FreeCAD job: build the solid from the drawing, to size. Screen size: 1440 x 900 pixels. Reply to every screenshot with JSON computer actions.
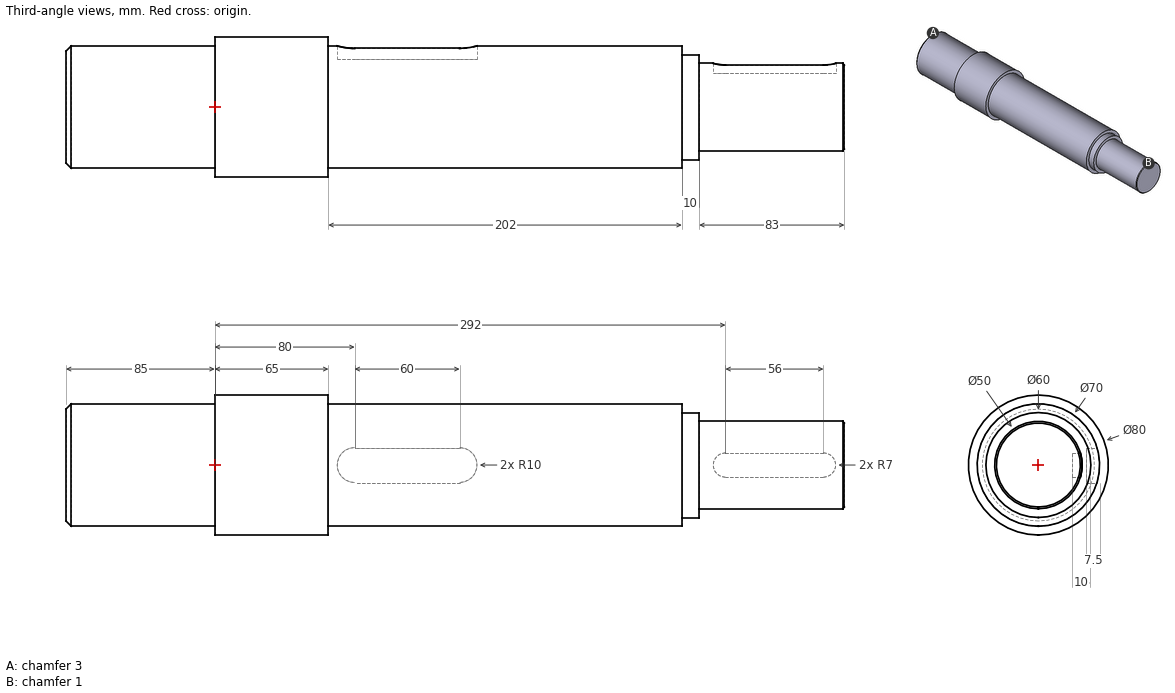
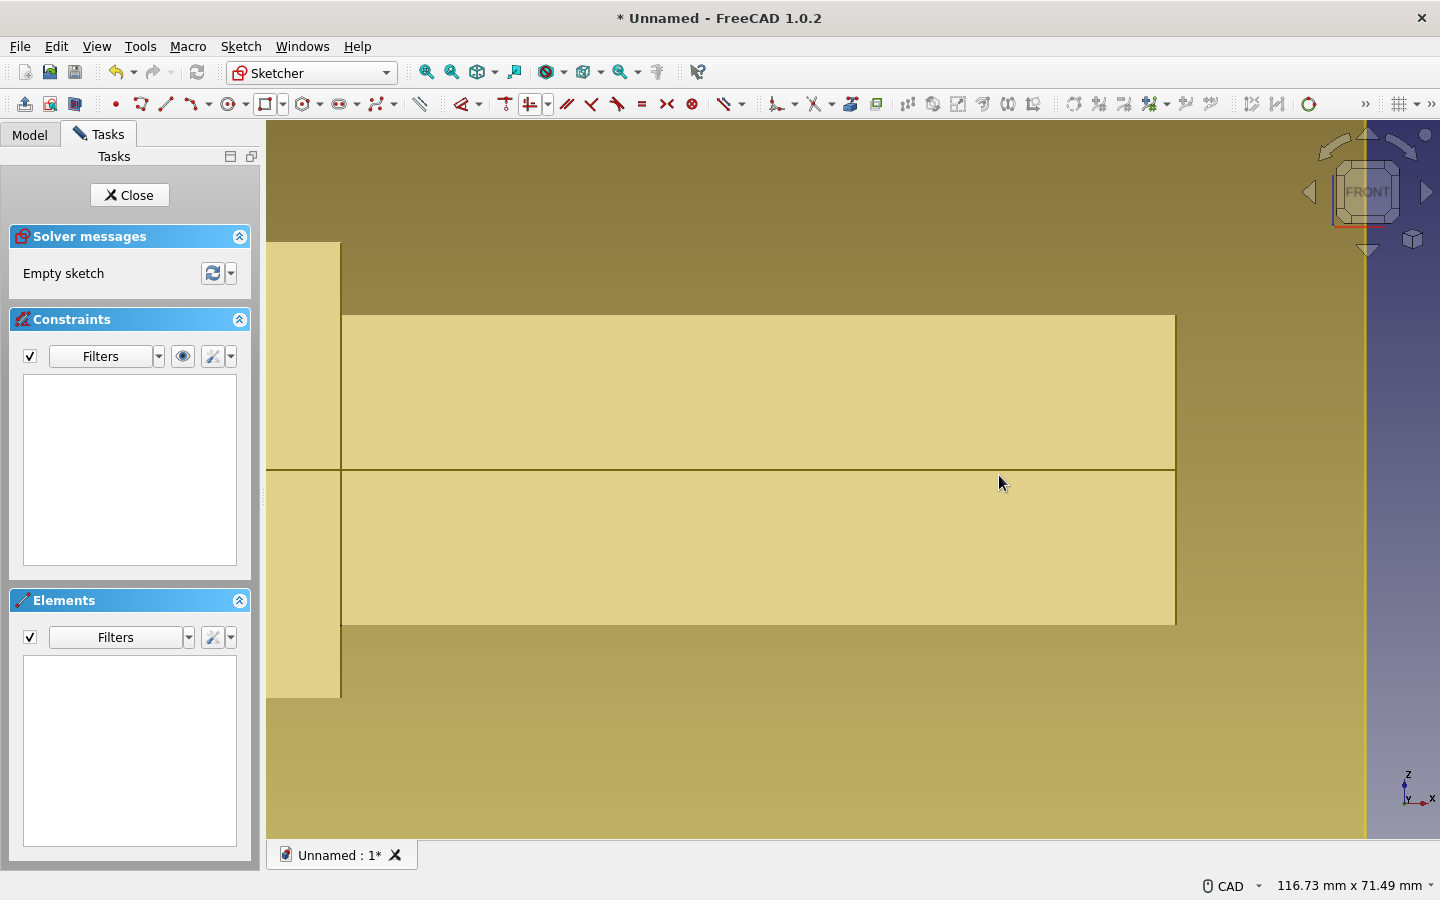
{"action": "key", "text": "g s"}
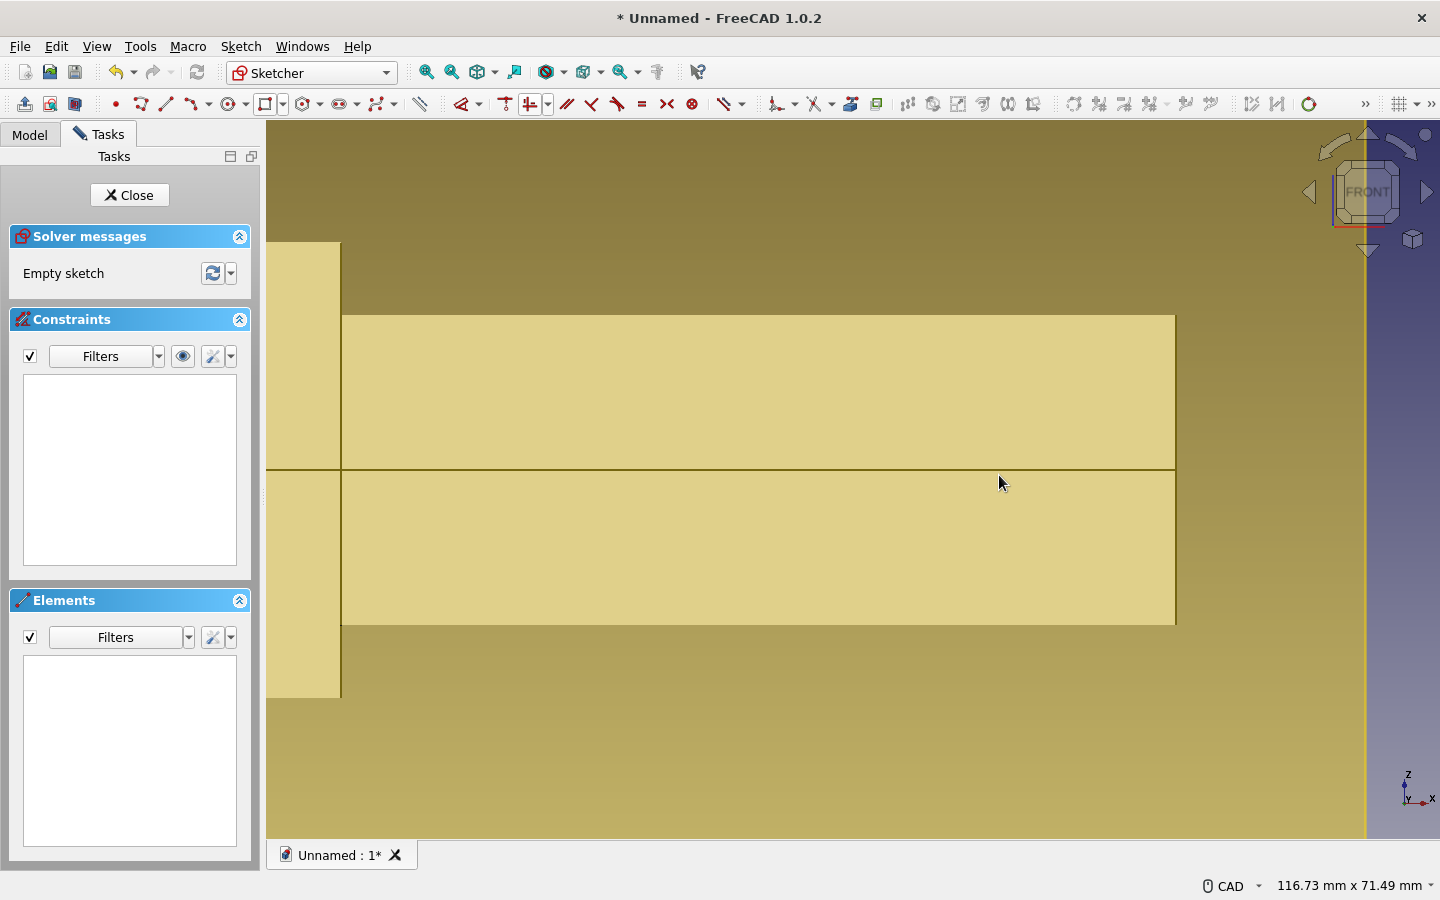
{"action": "left_click", "coordinate": [492, 470]}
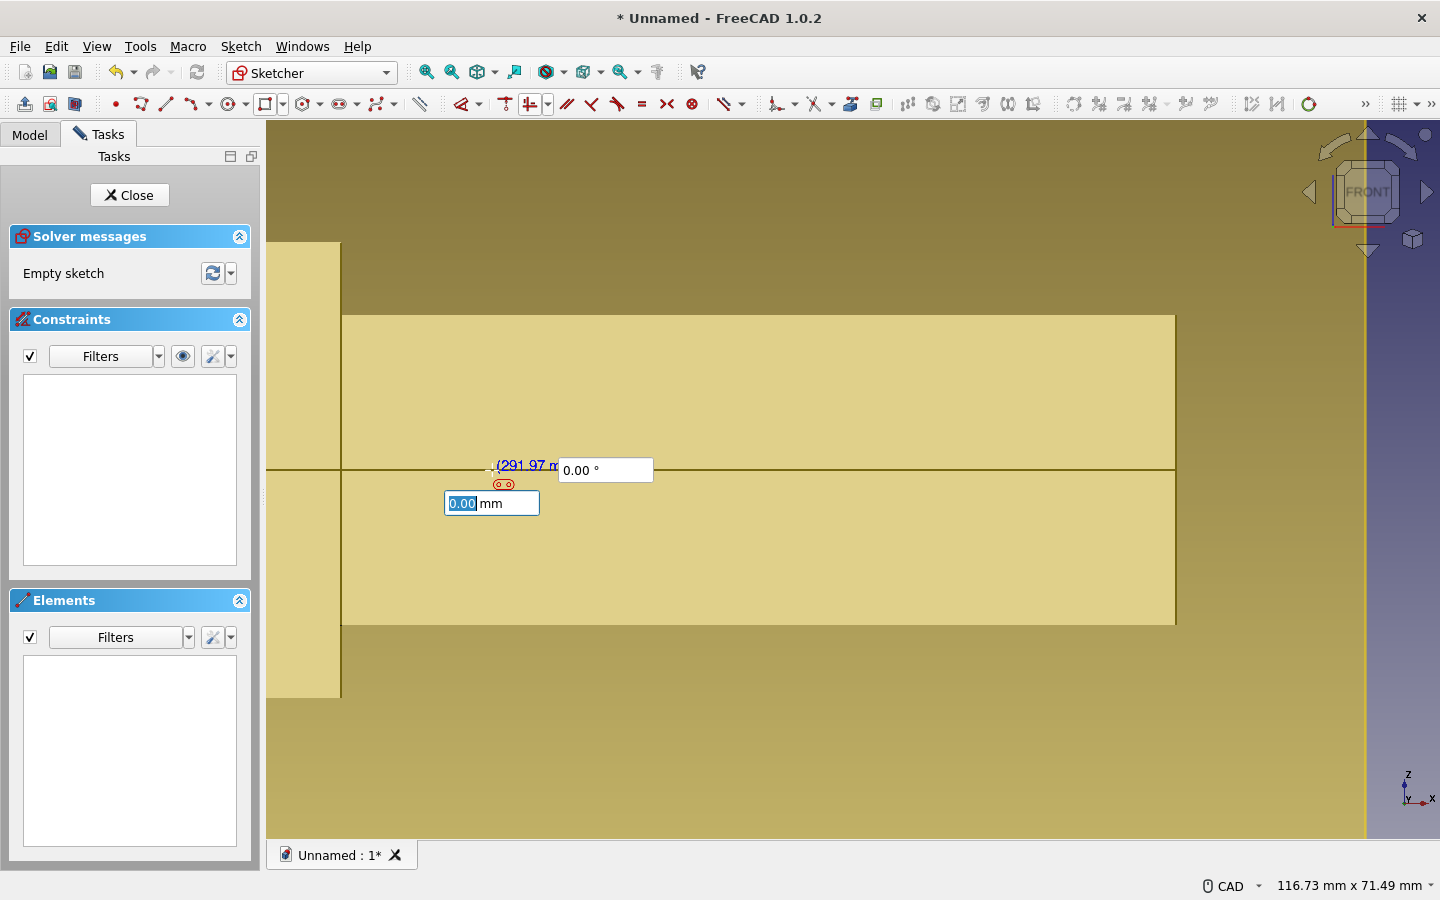
{"action": "left_click", "coordinate": [1055, 461]}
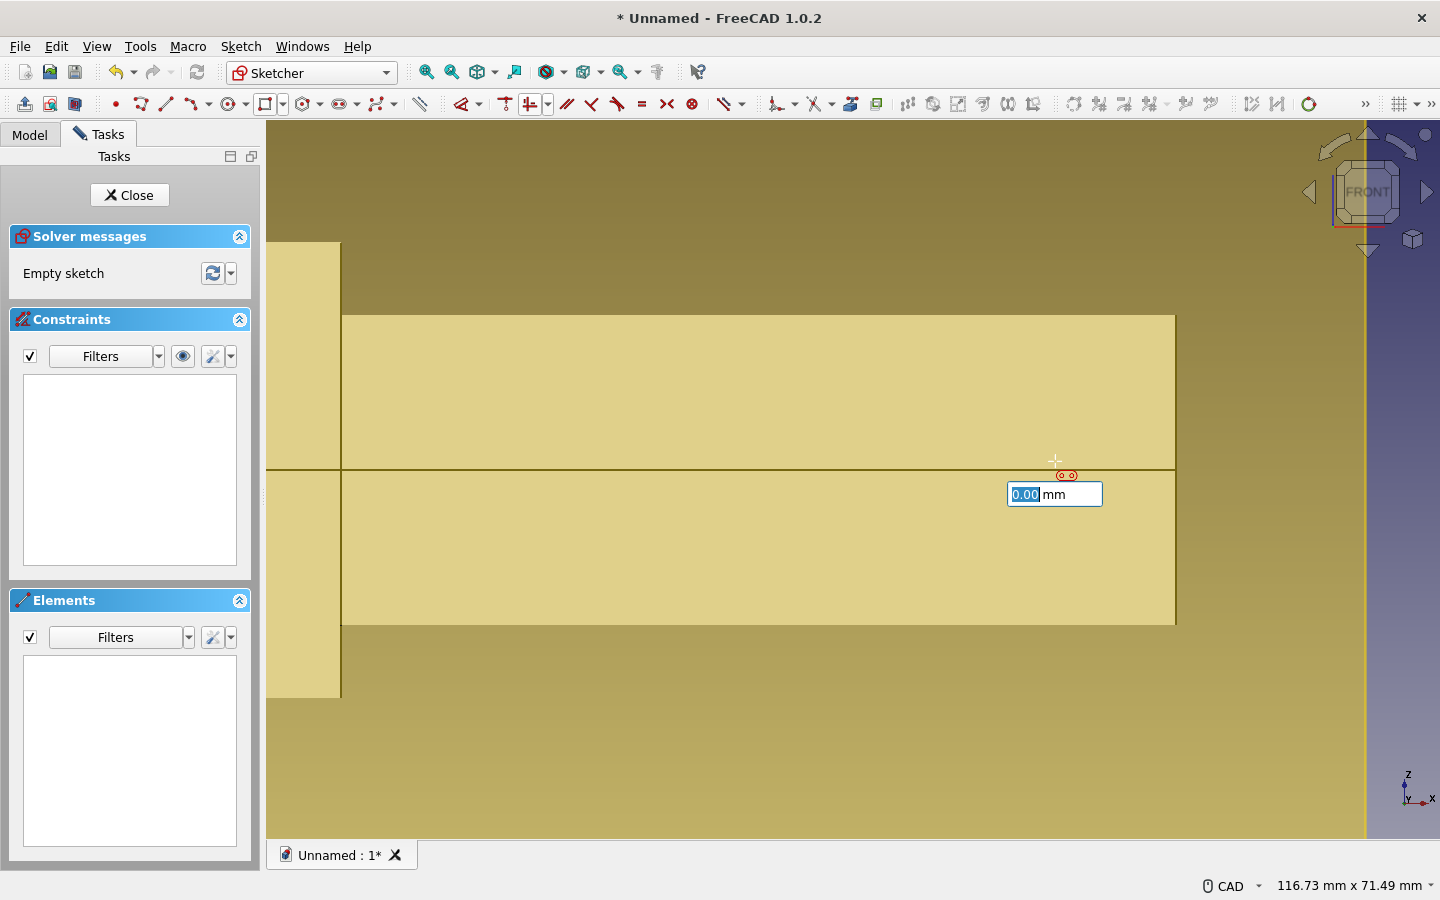
{"action": "left_click", "coordinate": [774, 400]}
{"action": "key", "text": "Escape"}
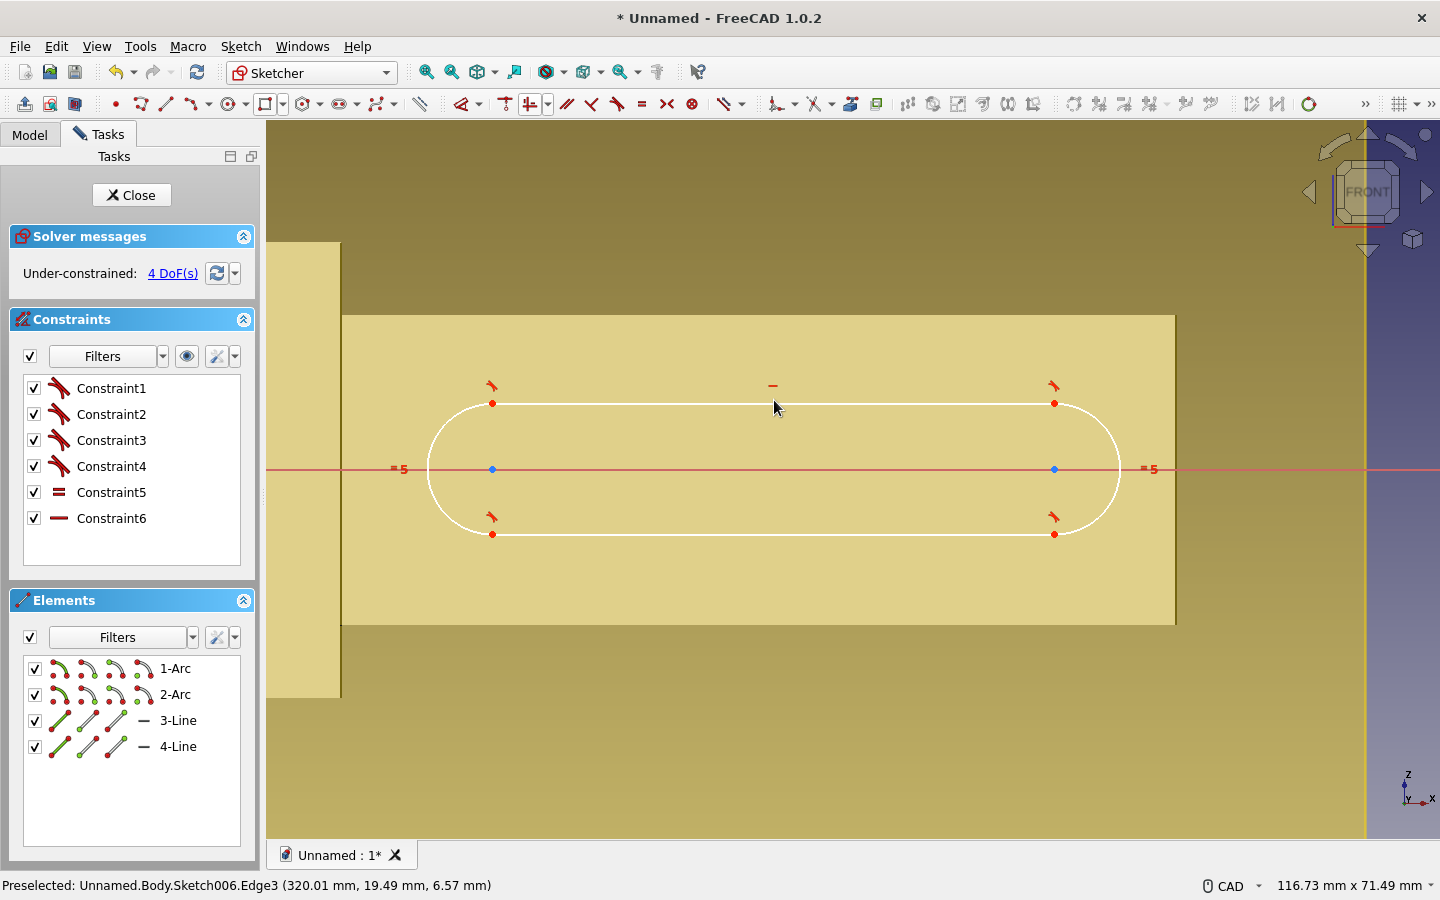
{"action": "left_click", "coordinate": [493, 469]}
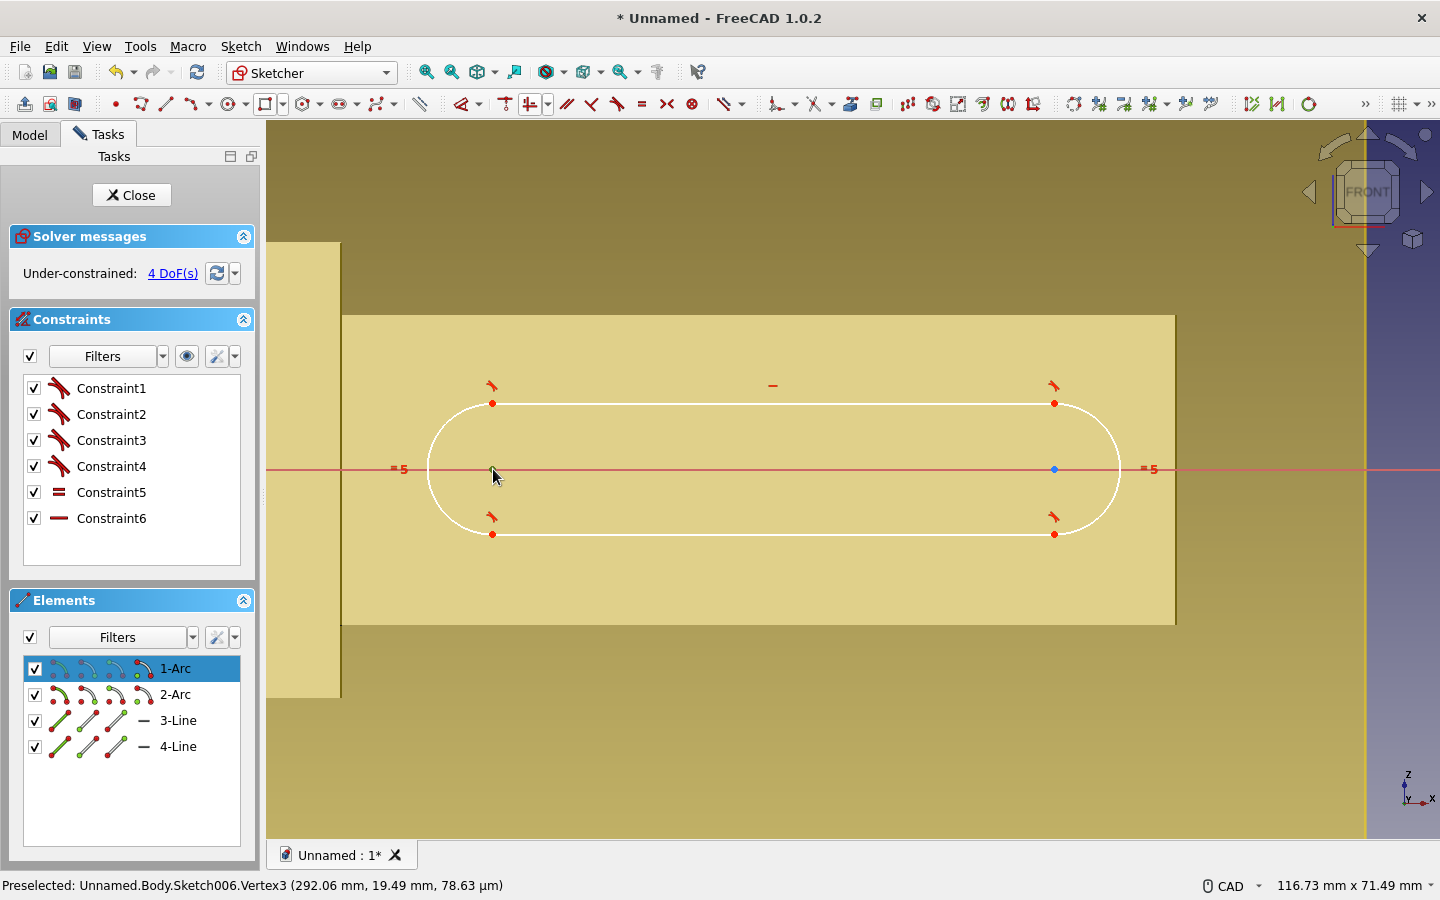
{"action": "left_click", "coordinate": [364, 470]}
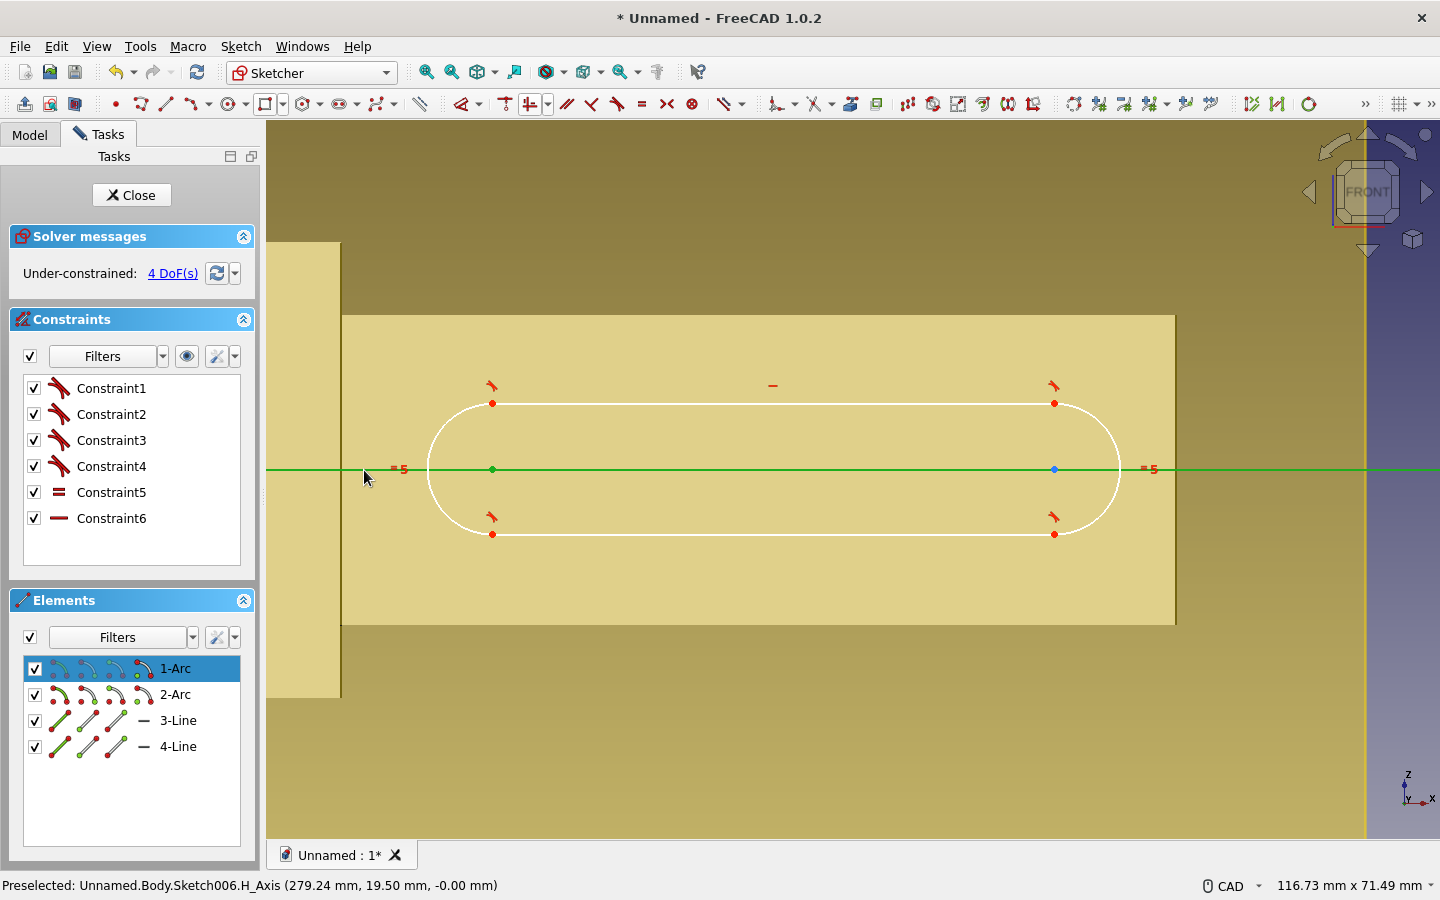
{"action": "left_click", "coordinate": [505, 104]}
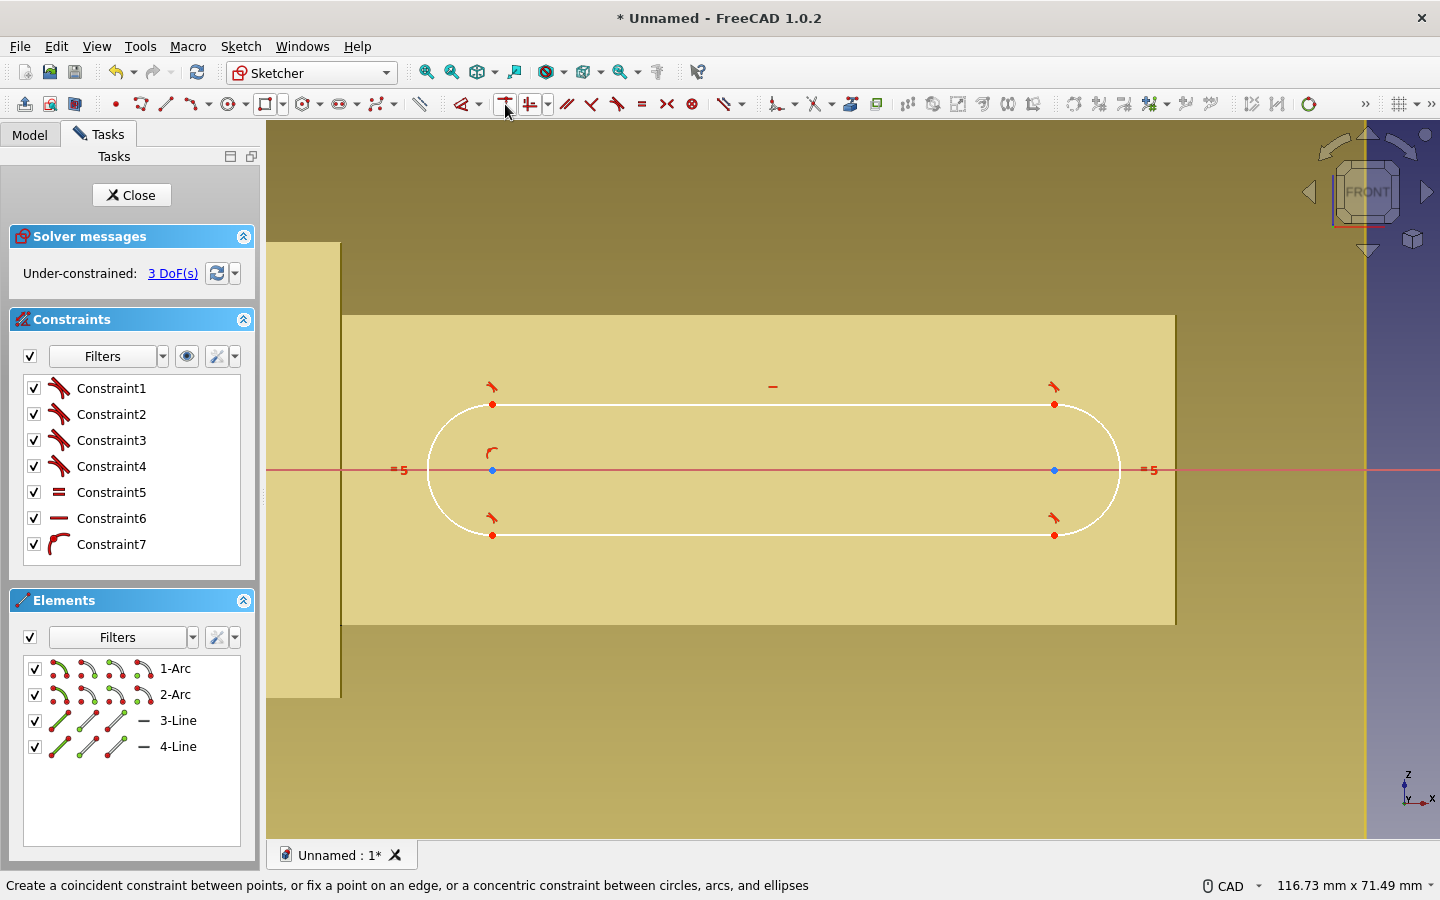
{"action": "key", "text": "d"}